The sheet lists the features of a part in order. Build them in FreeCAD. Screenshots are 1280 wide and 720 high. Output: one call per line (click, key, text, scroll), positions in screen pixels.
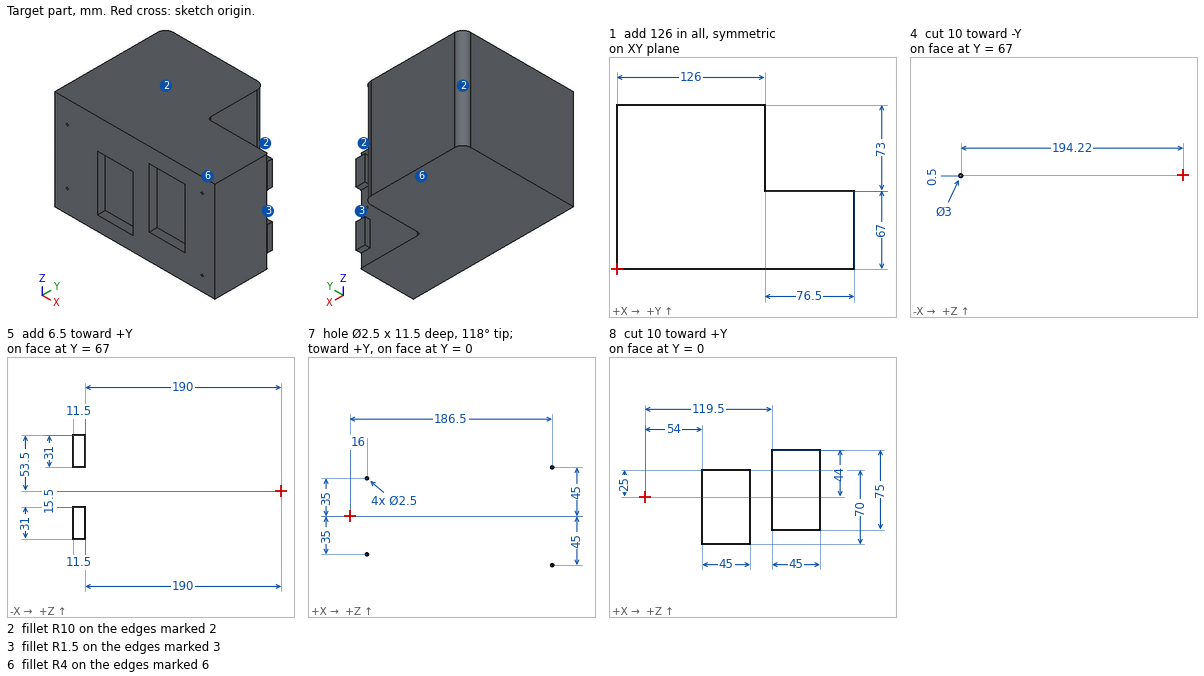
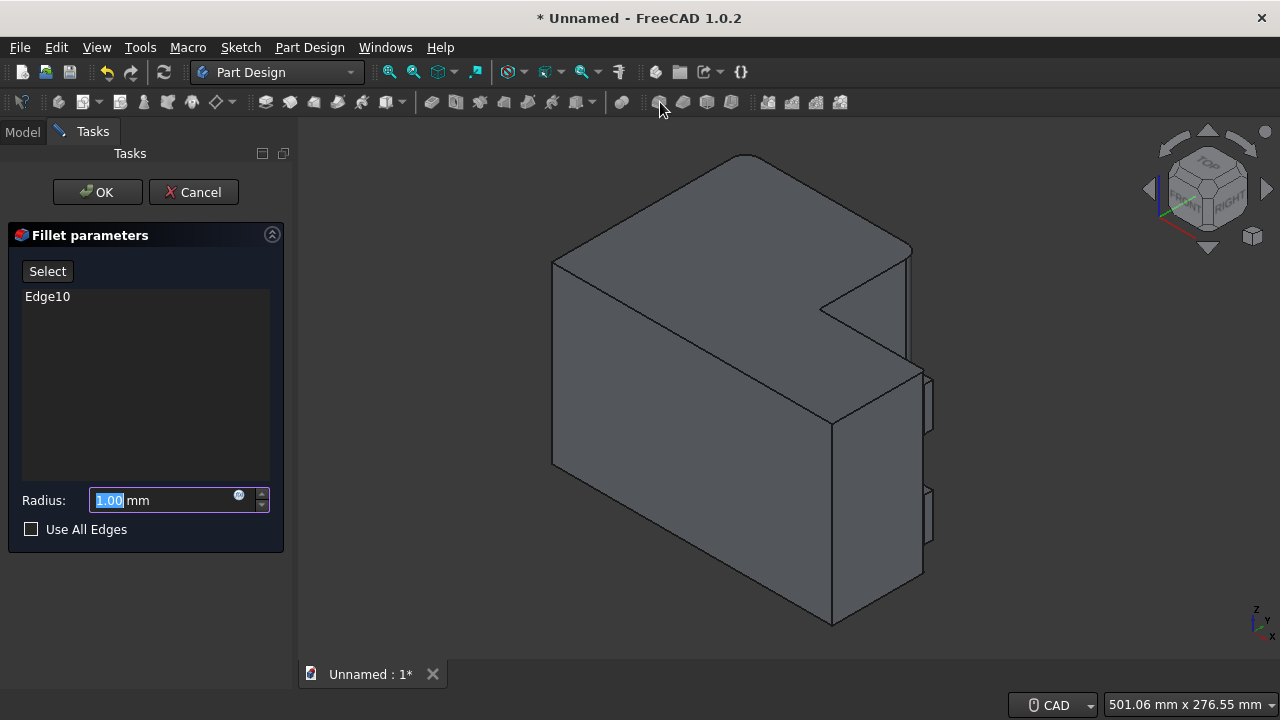
text(4)
key(Tab)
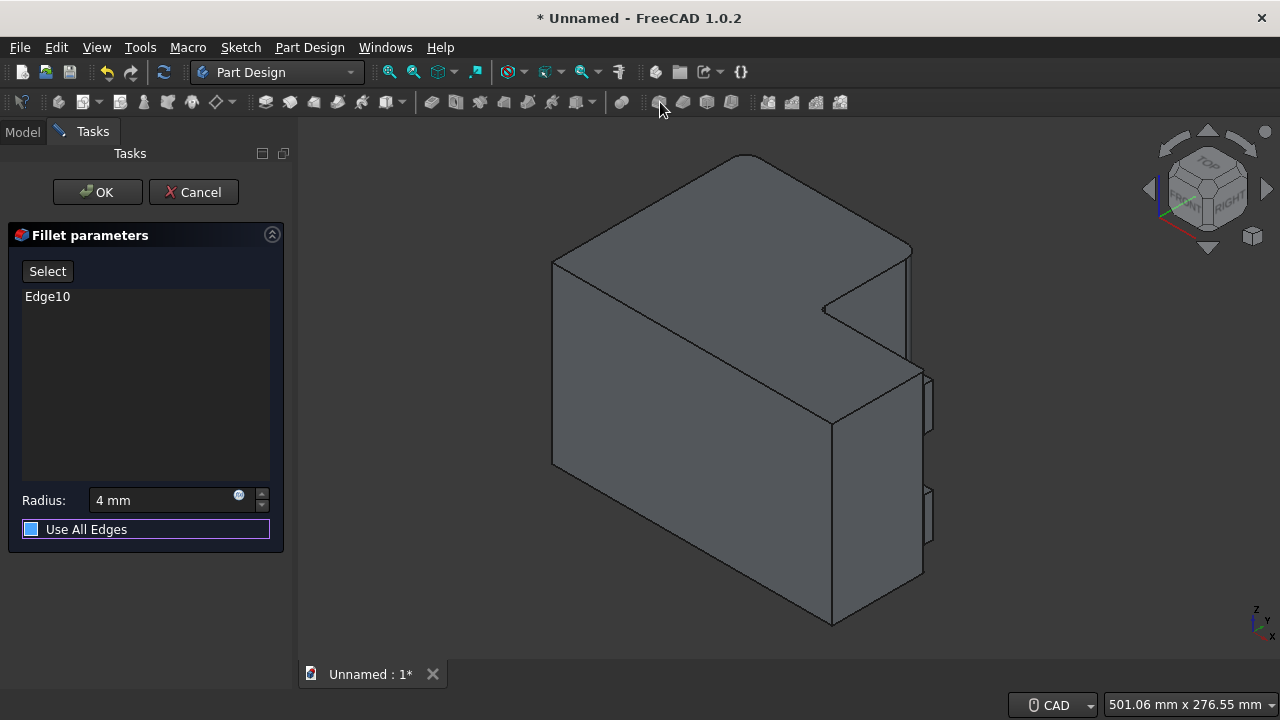
click(98, 192)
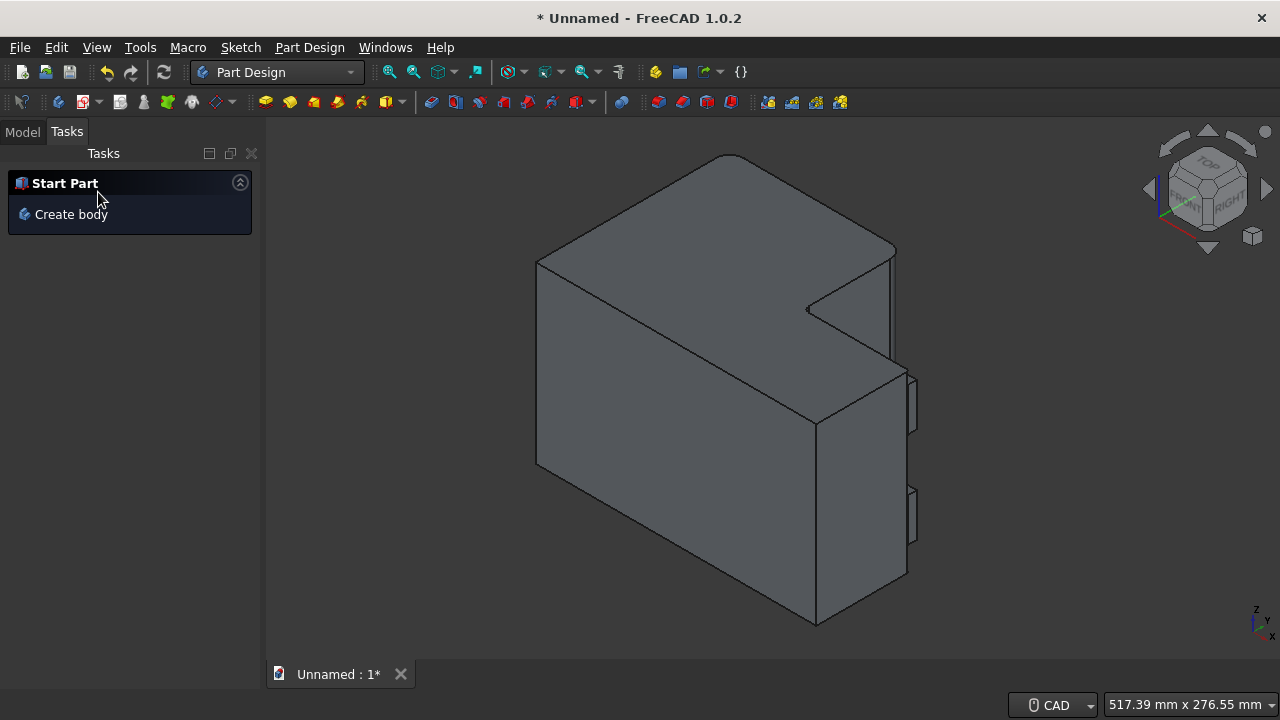
click(716, 466)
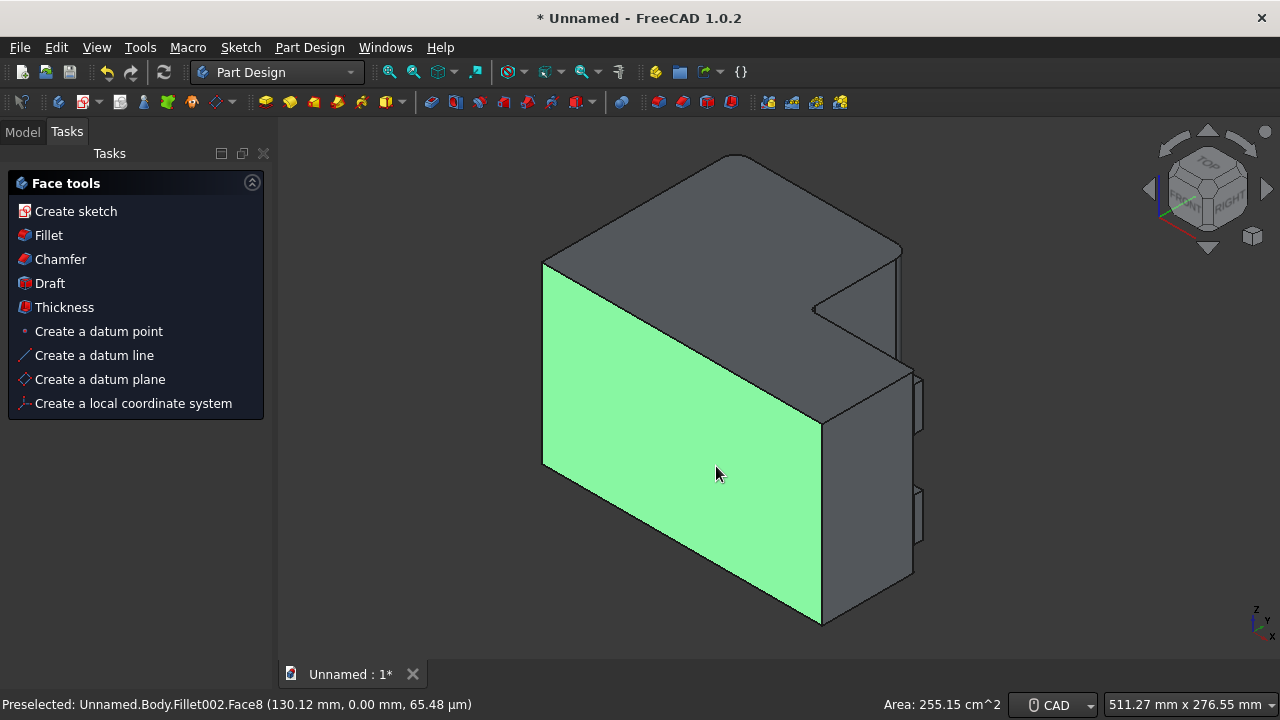
click(84, 102)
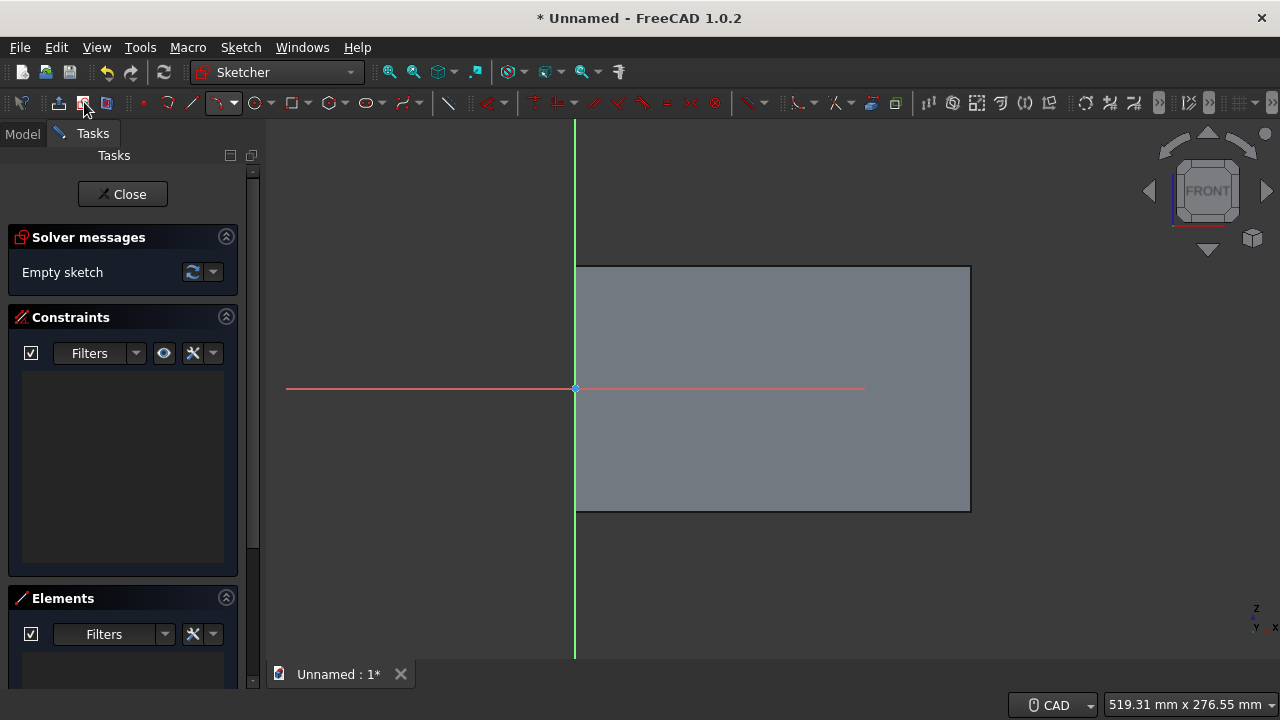
scroll(869, 389, up, 2)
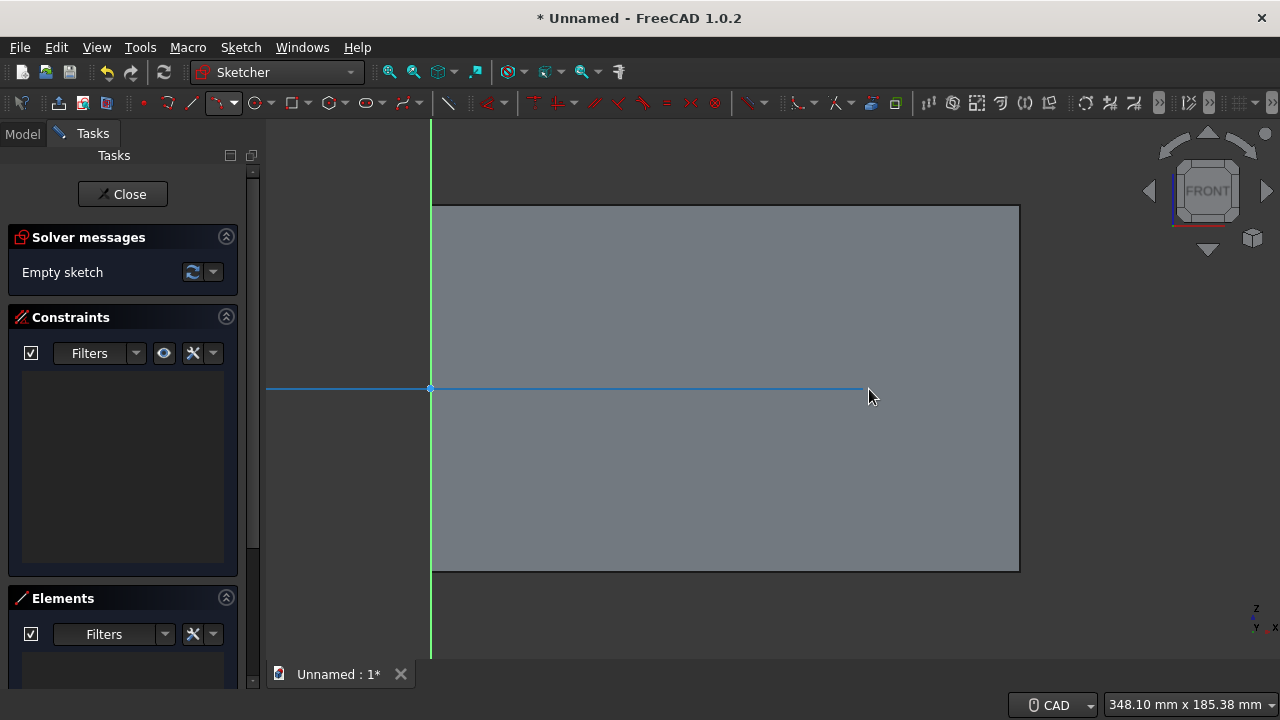
key(g)
key(c)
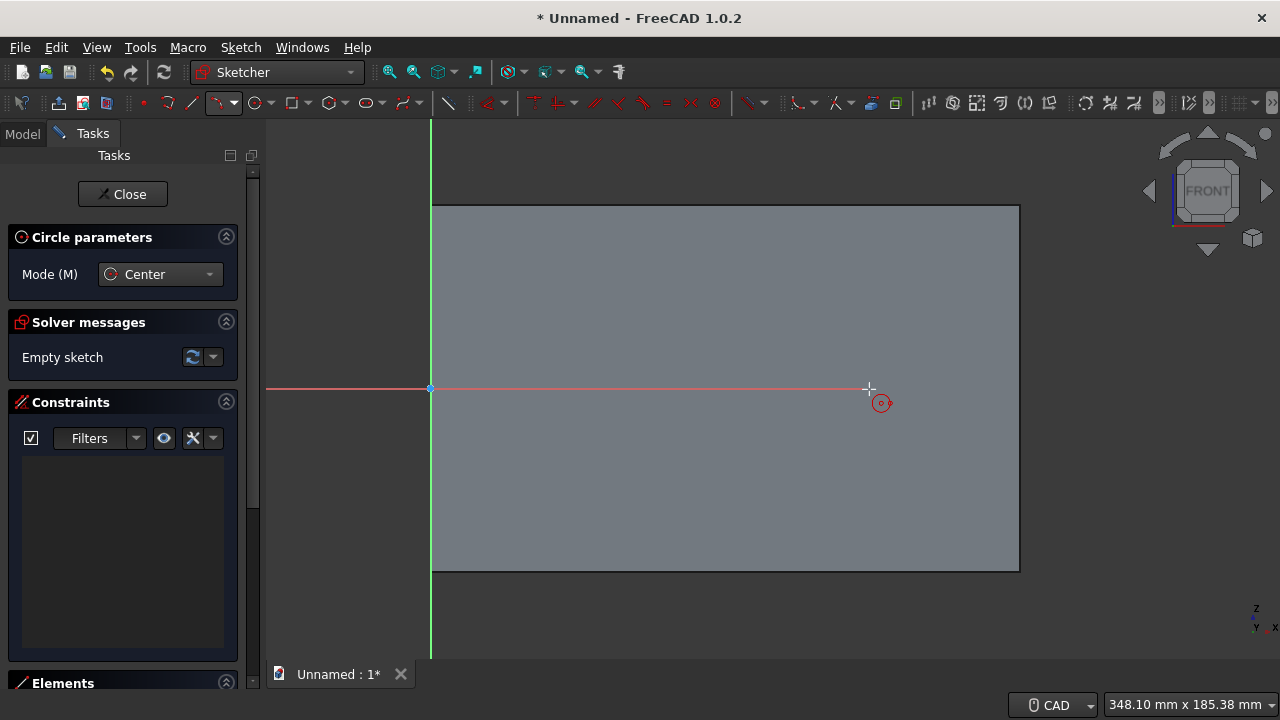
scroll(477, 287, up, 10)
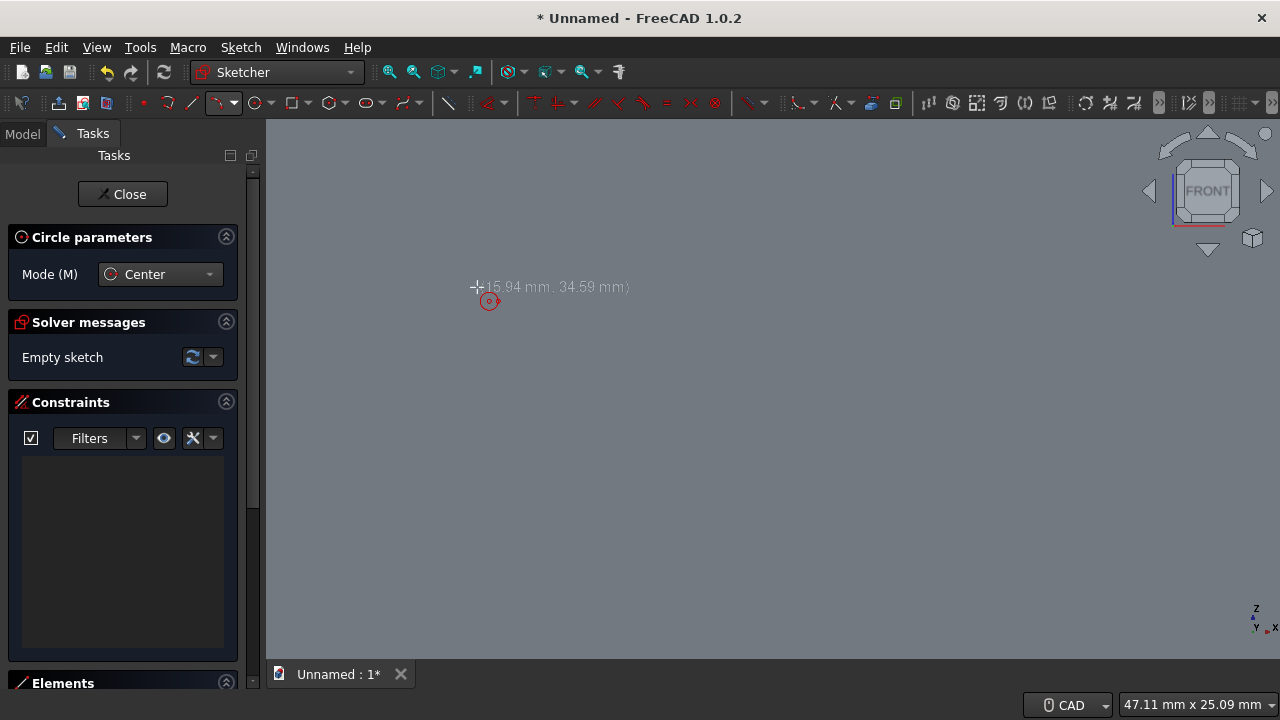
scroll(478, 288, down, 10)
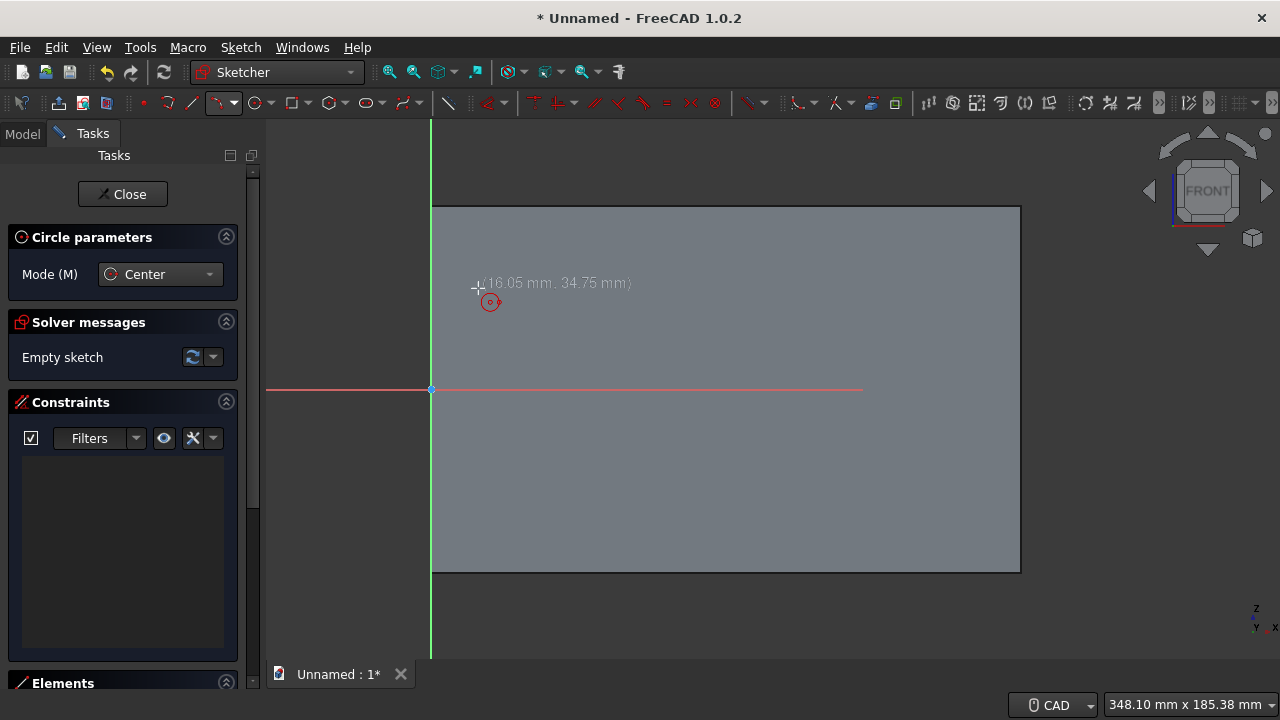
click(478, 288)
move(481, 285)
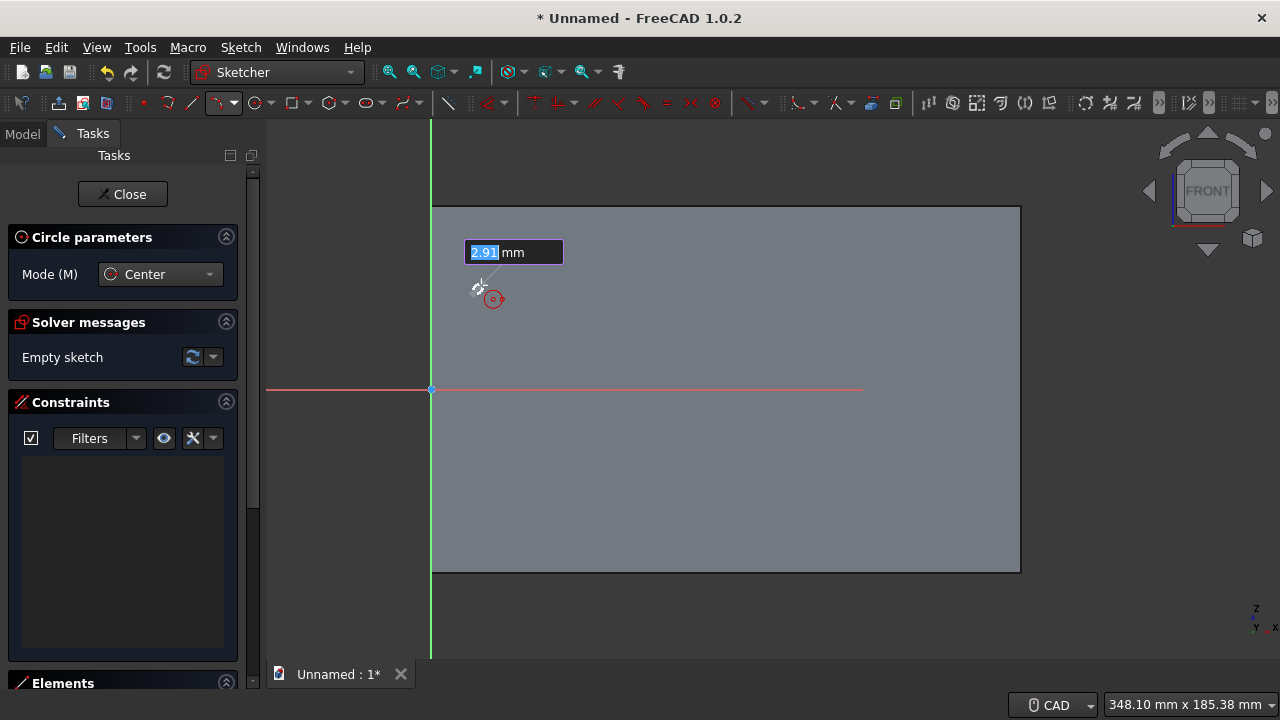
text(2.5)
key(Return)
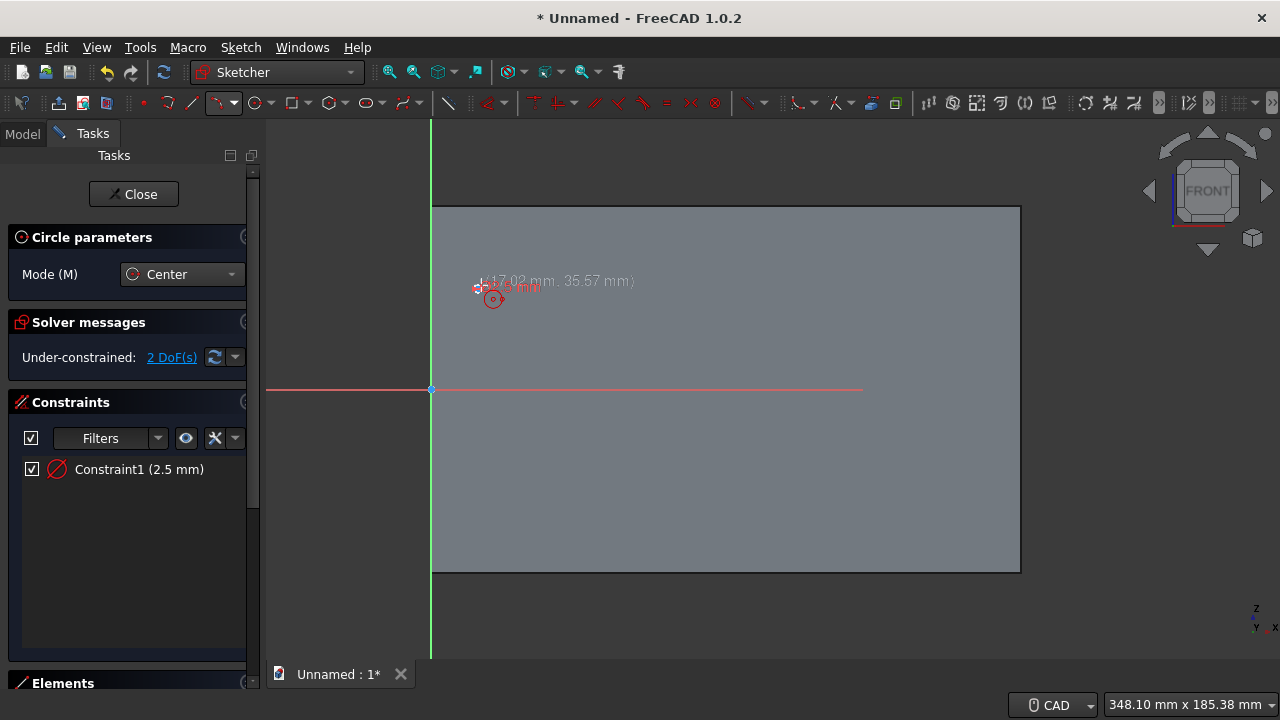
scroll(478, 492, up, 10)